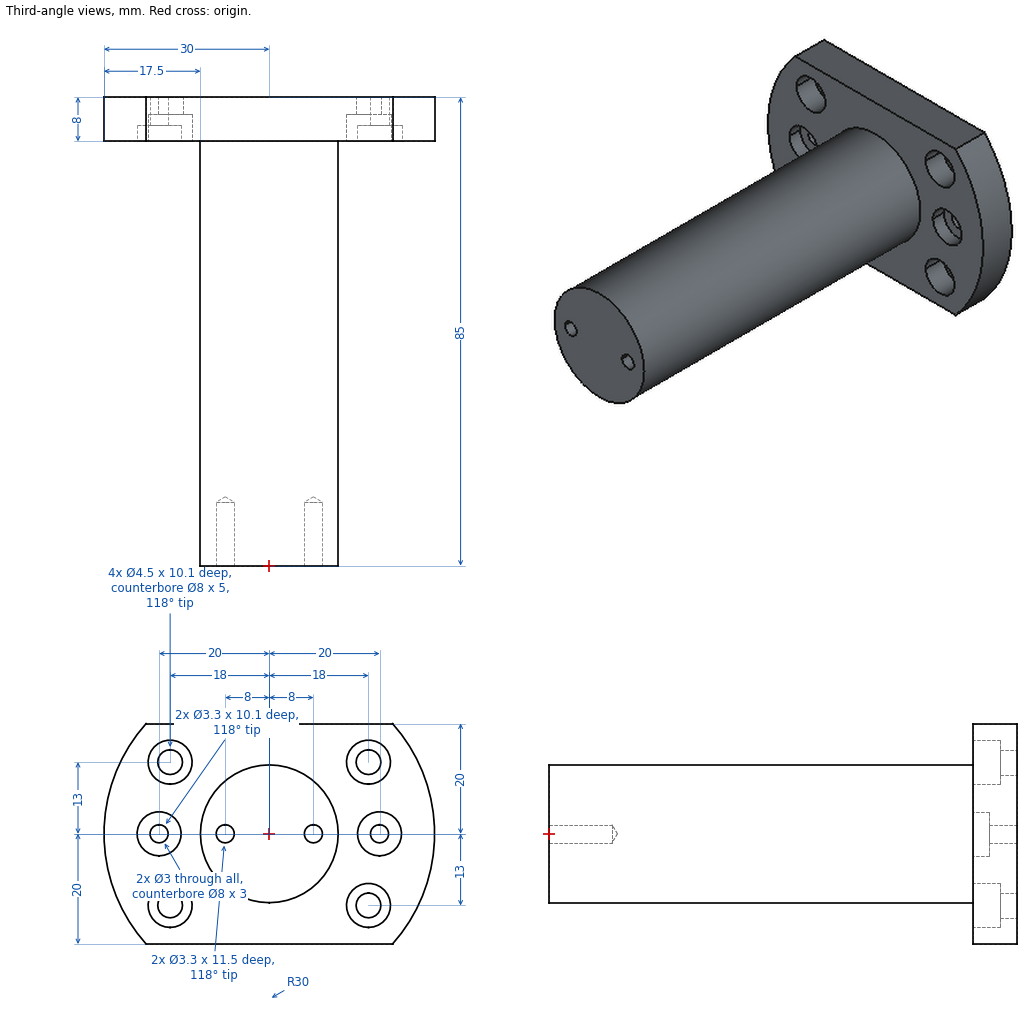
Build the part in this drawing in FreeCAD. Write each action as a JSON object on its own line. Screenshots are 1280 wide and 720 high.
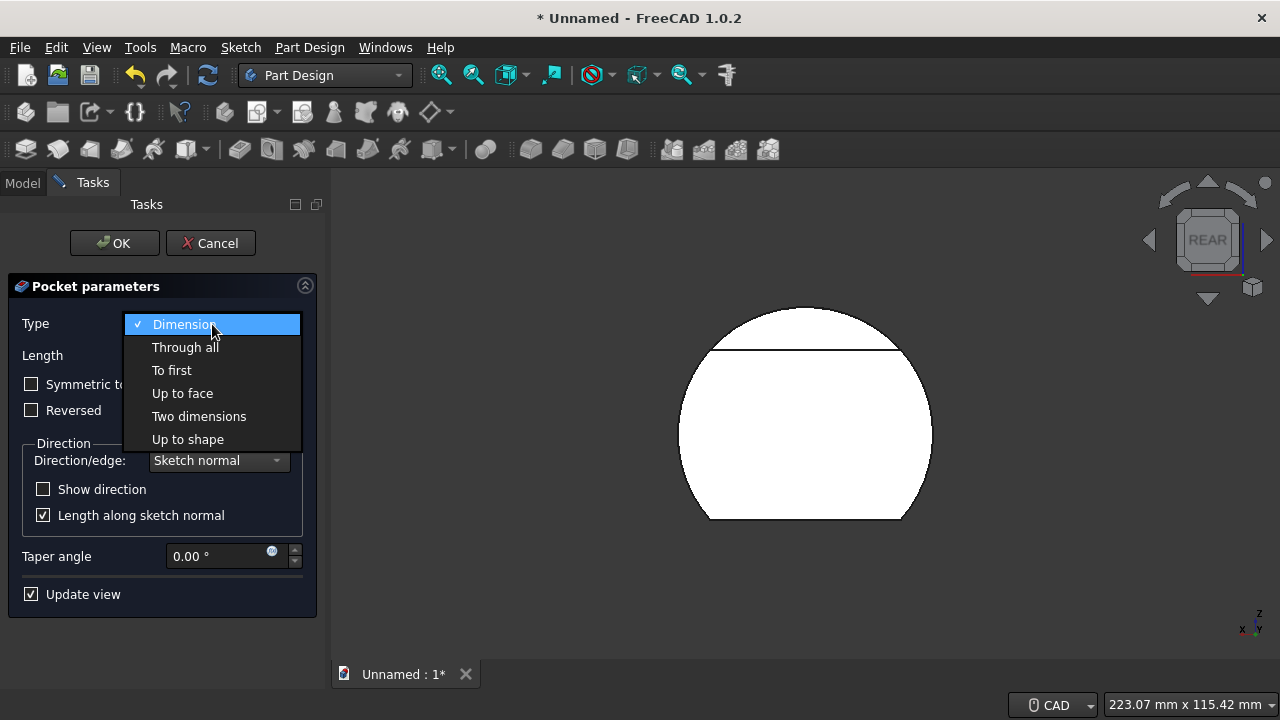
{"action": "left_click", "coordinate": [212, 370]}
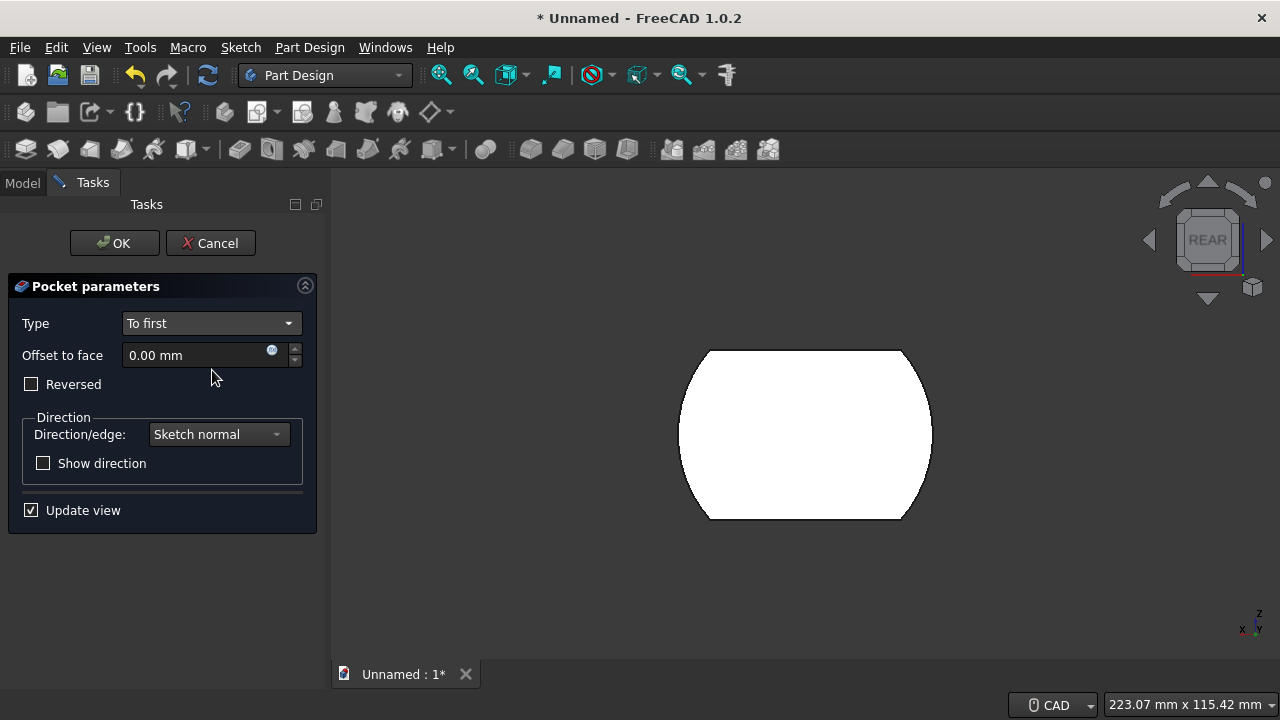
{"action": "left_click", "coordinate": [115, 243]}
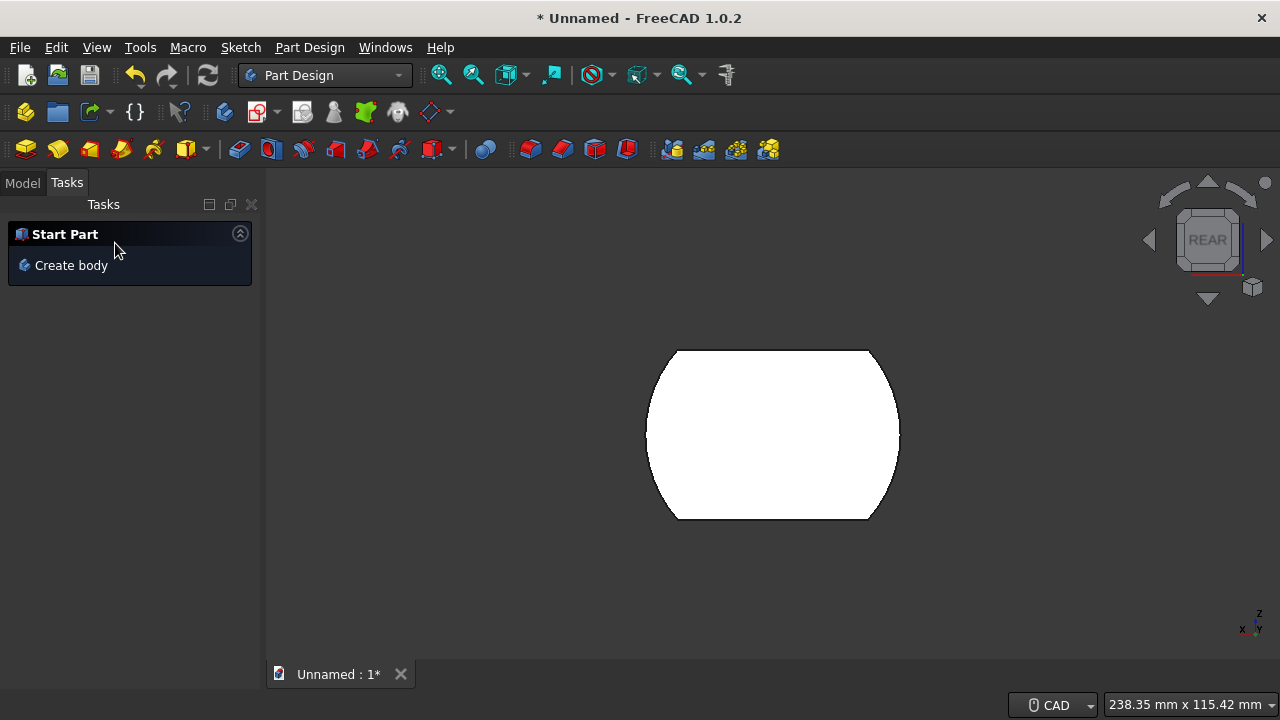
{"action": "left_click", "coordinate": [442, 76]}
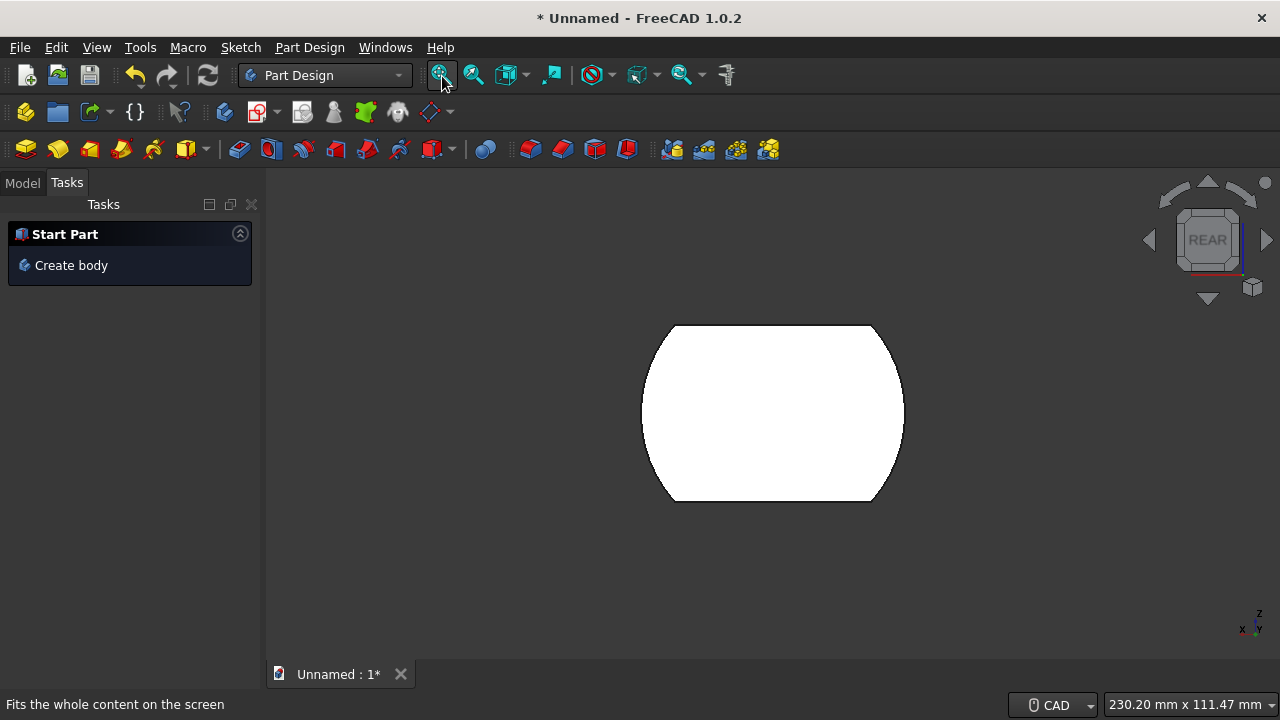
{"action": "key", "text": "0"}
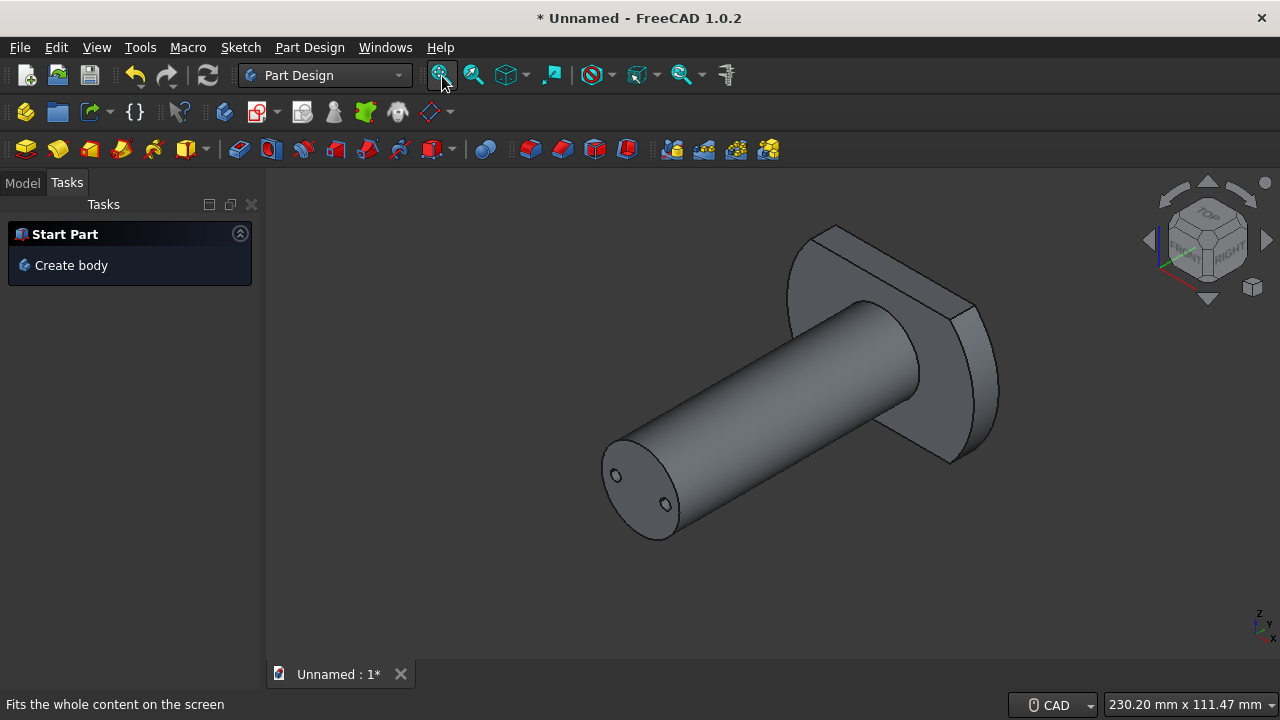
{"action": "left_click", "coordinate": [934, 422]}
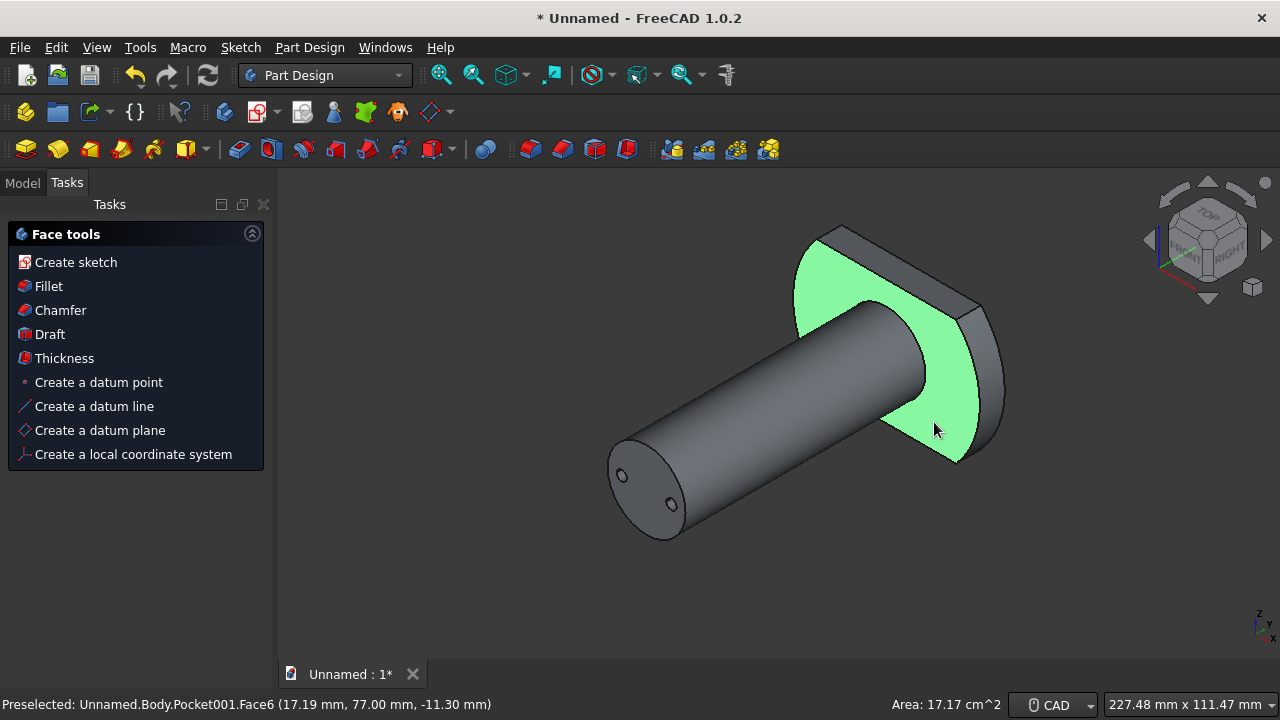
{"action": "left_click", "coordinate": [258, 112]}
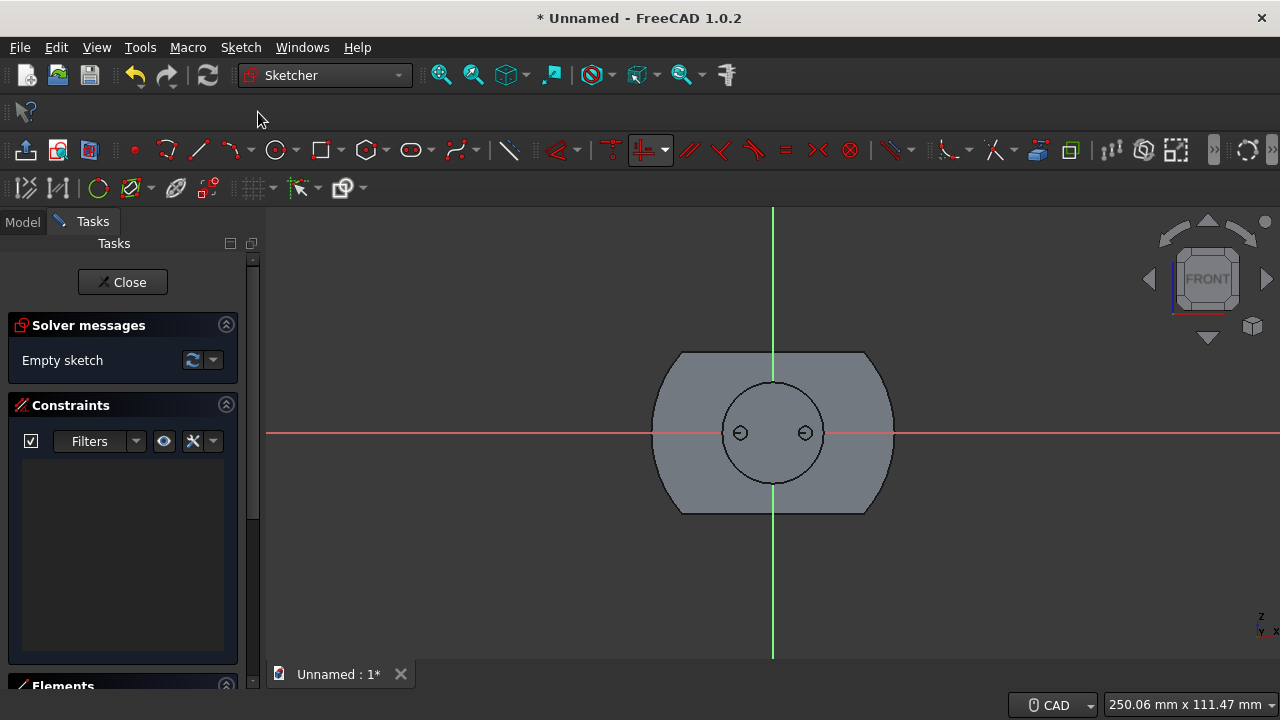
{"action": "scroll", "coordinate": [803, 433], "scroll_direction": "up", "scroll_amount": 6}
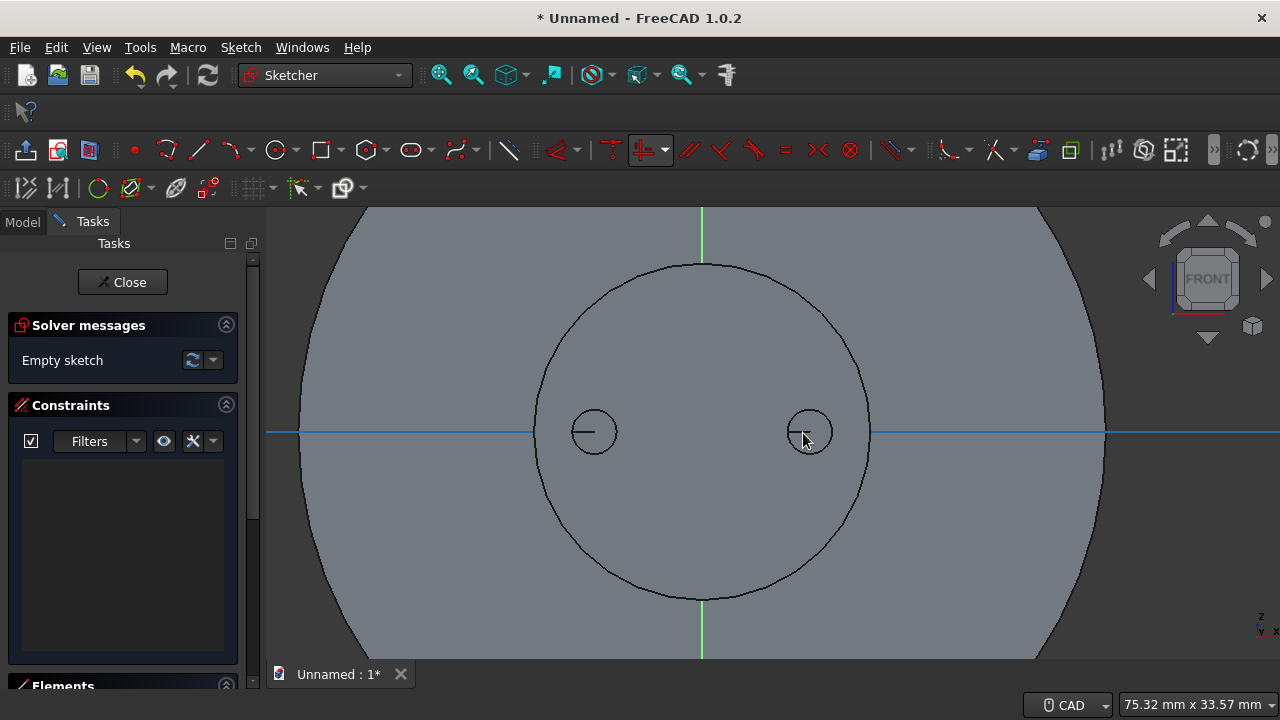
{"action": "left_click", "coordinate": [276, 150]}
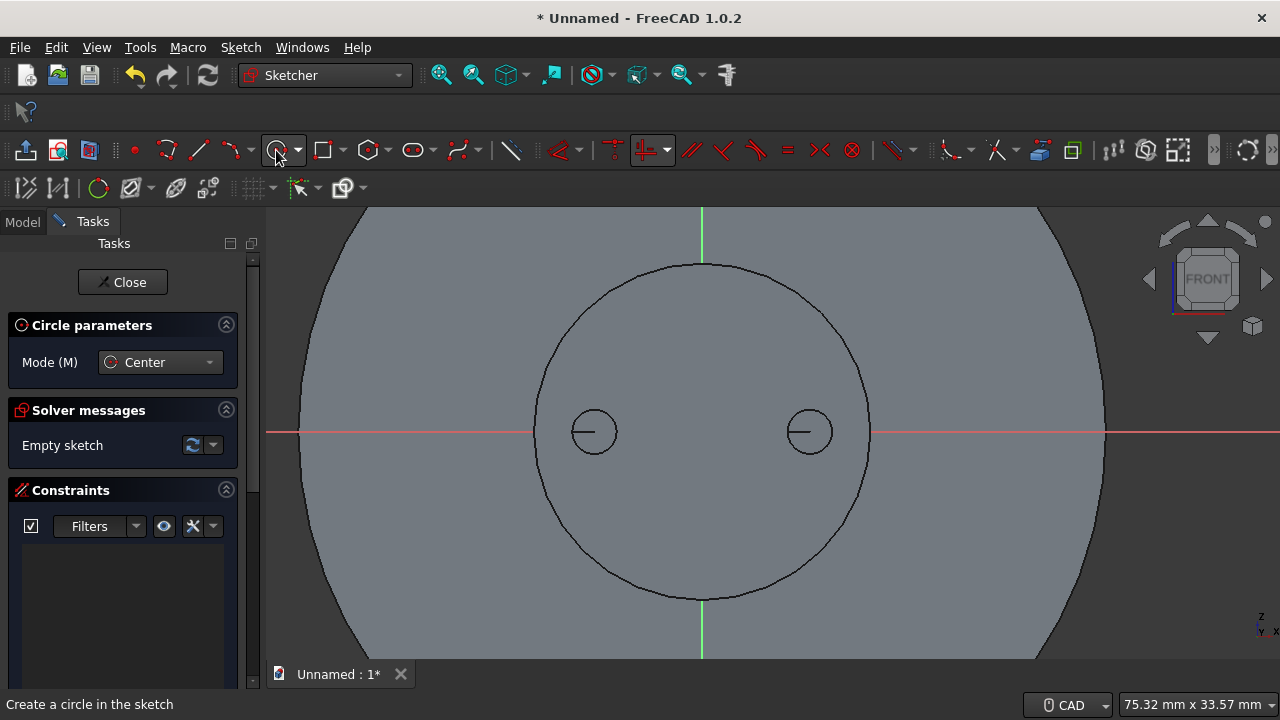
{"action": "left_click", "coordinate": [433, 432]}
{"action": "mouse_move", "coordinate": [447, 418]}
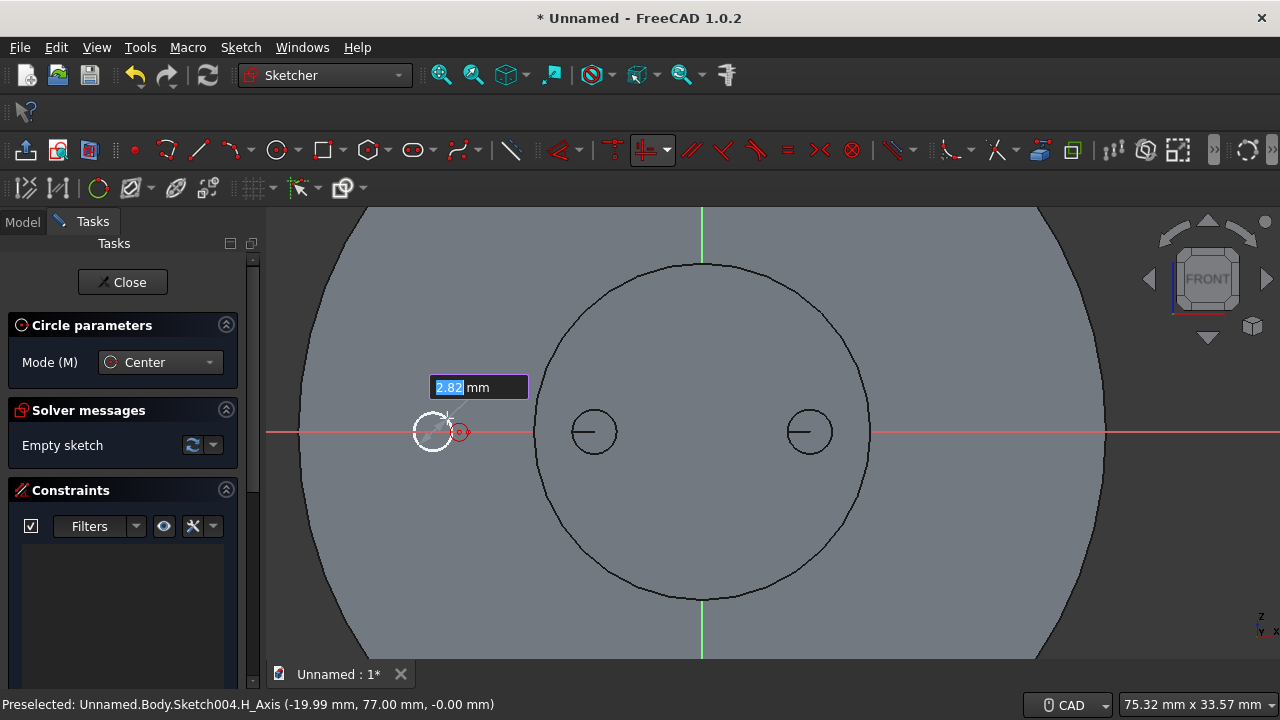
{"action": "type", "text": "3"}
{"action": "key", "text": "Return"}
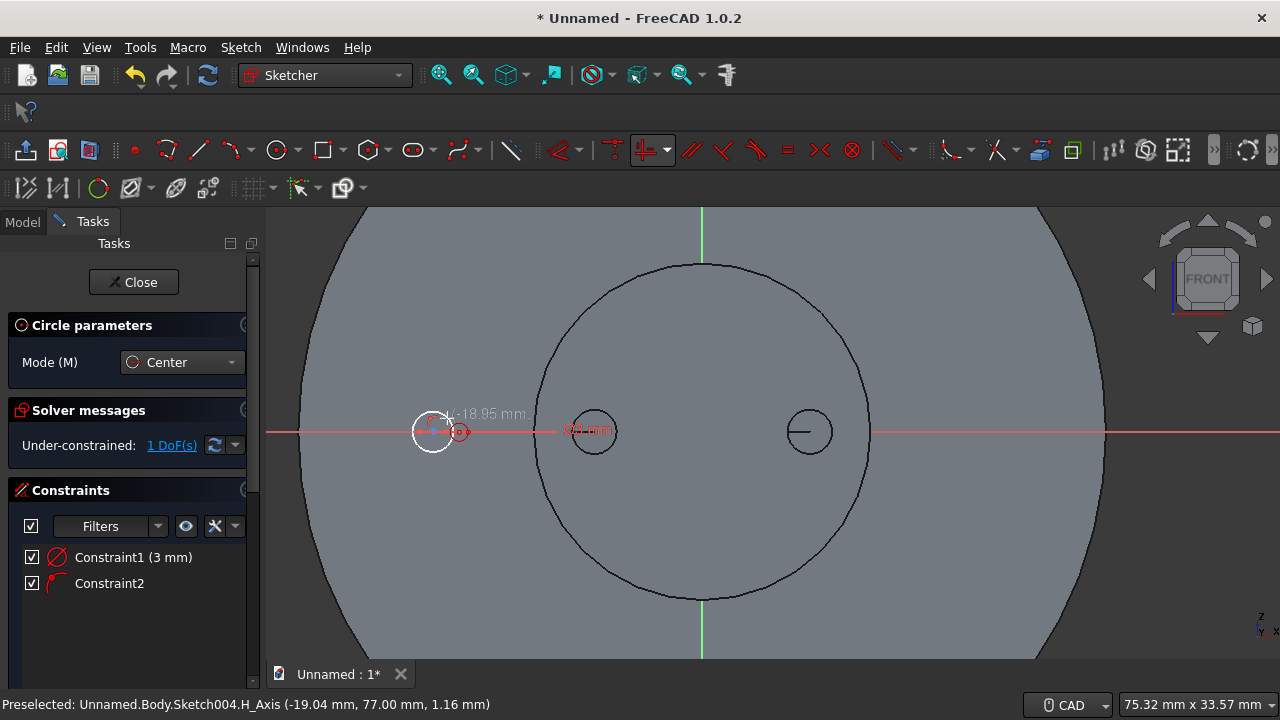
{"action": "left_click", "coordinate": [971, 432]}
{"action": "mouse_move", "coordinate": [986, 418]}